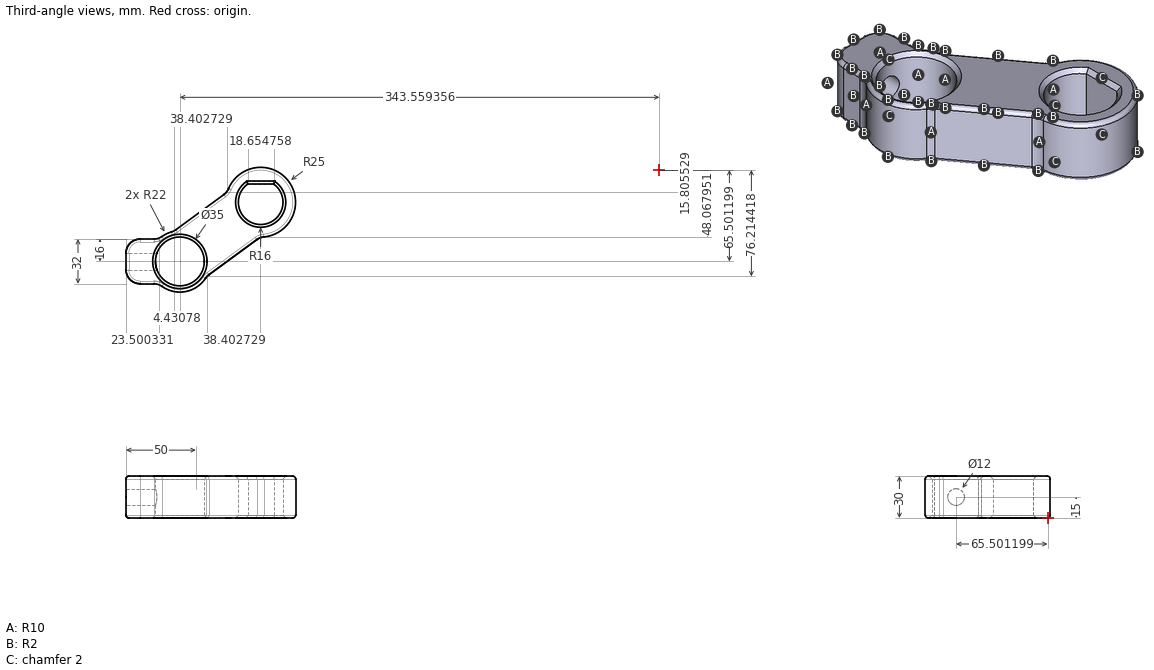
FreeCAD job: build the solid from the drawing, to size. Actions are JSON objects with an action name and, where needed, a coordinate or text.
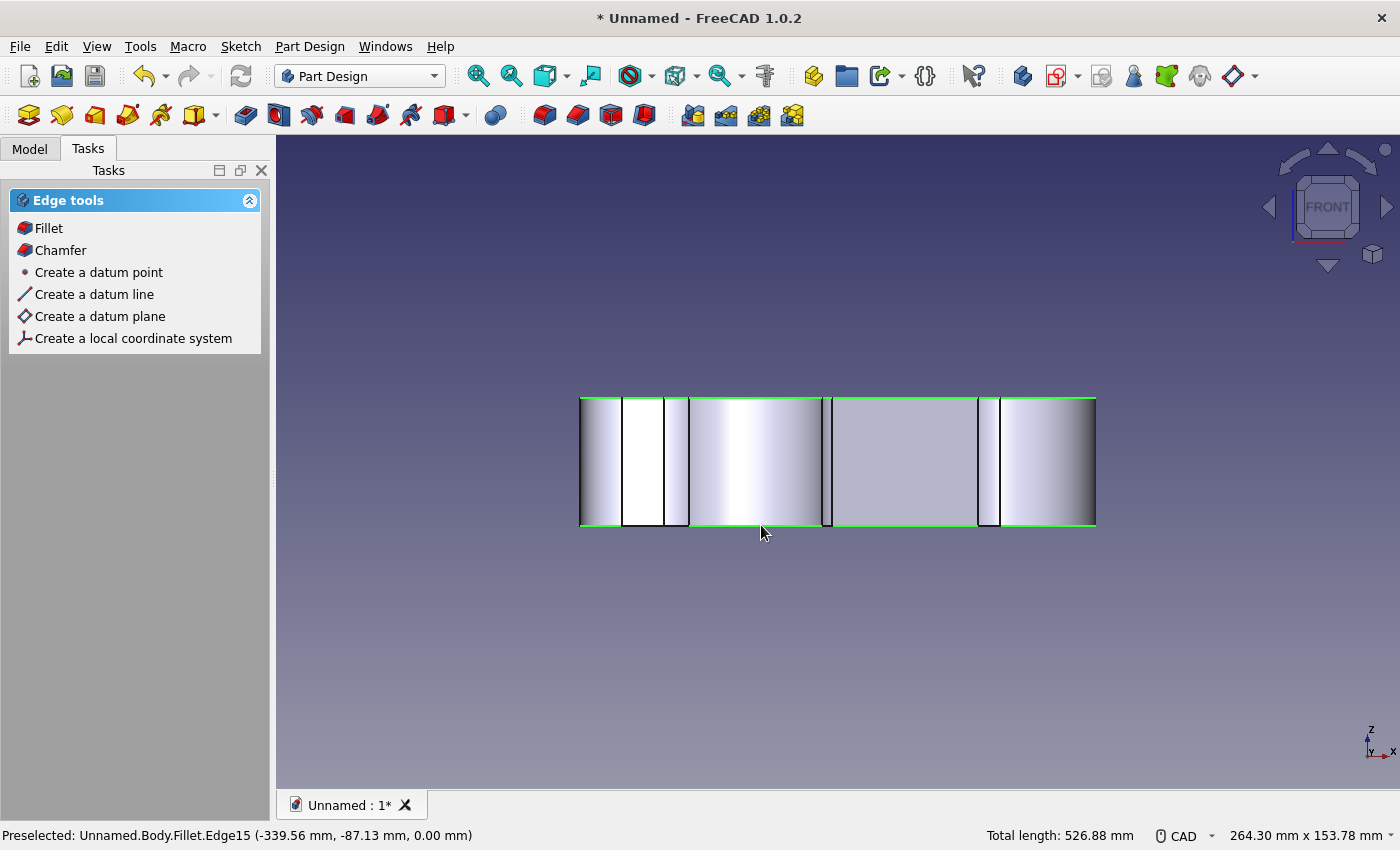
{"action": "left_click", "coordinate": [643, 525], "text": "ctrl"}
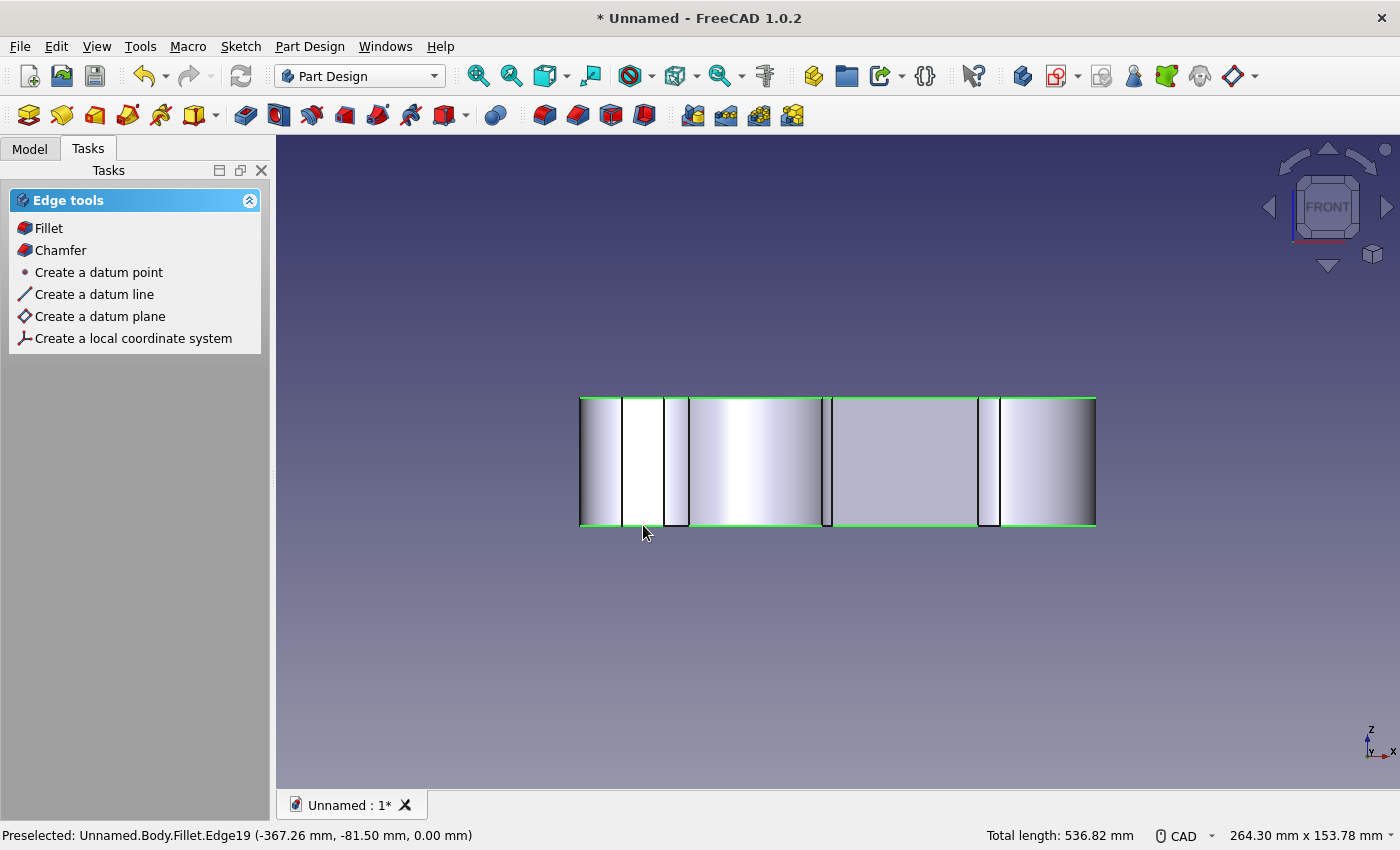
{"action": "left_click", "coordinate": [828, 525], "text": "ctrl"}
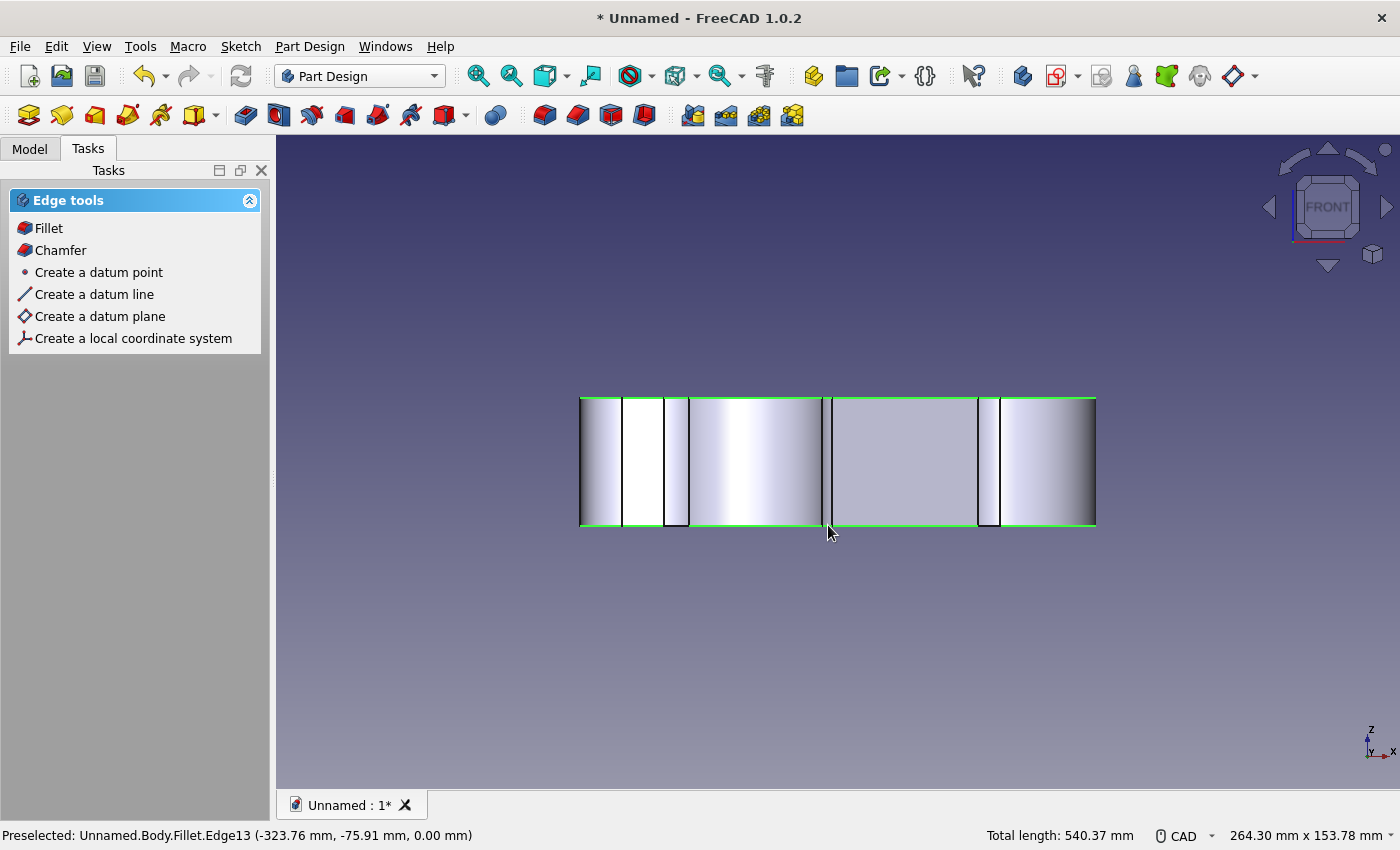
{"action": "left_click", "coordinate": [678, 525], "text": "ctrl"}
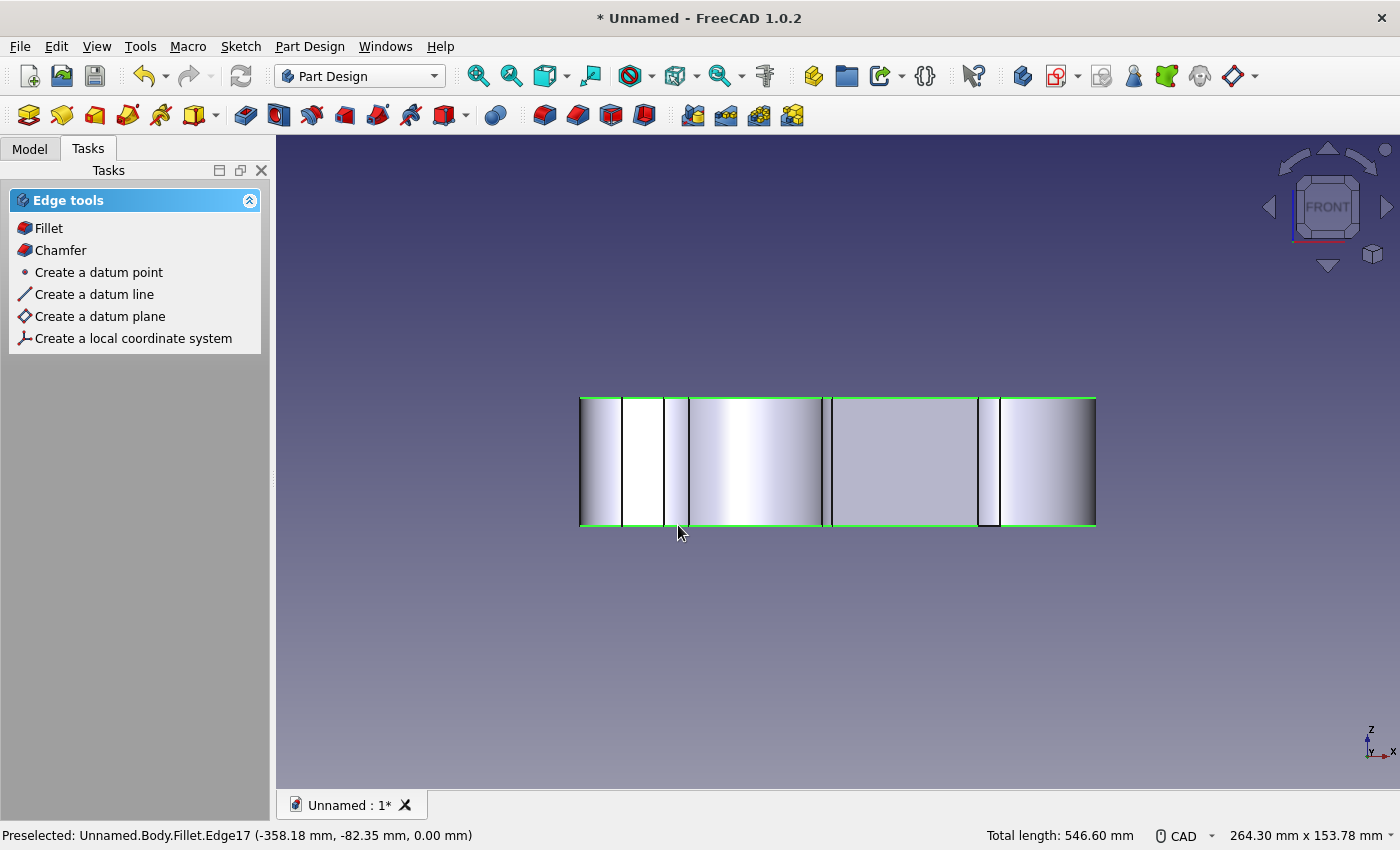
{"action": "left_click", "coordinate": [989, 525], "text": "ctrl"}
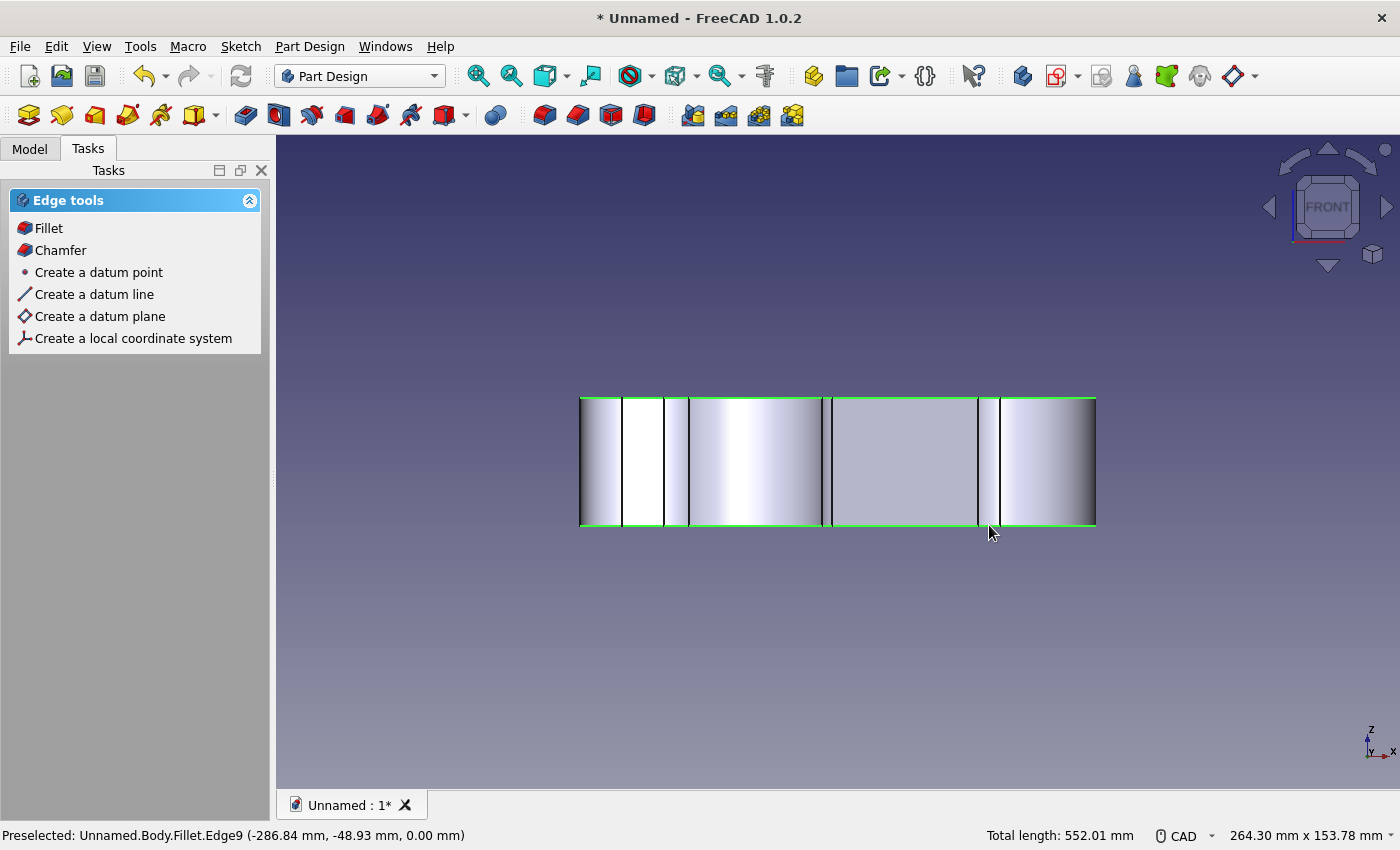
{"action": "key", "text": "3"}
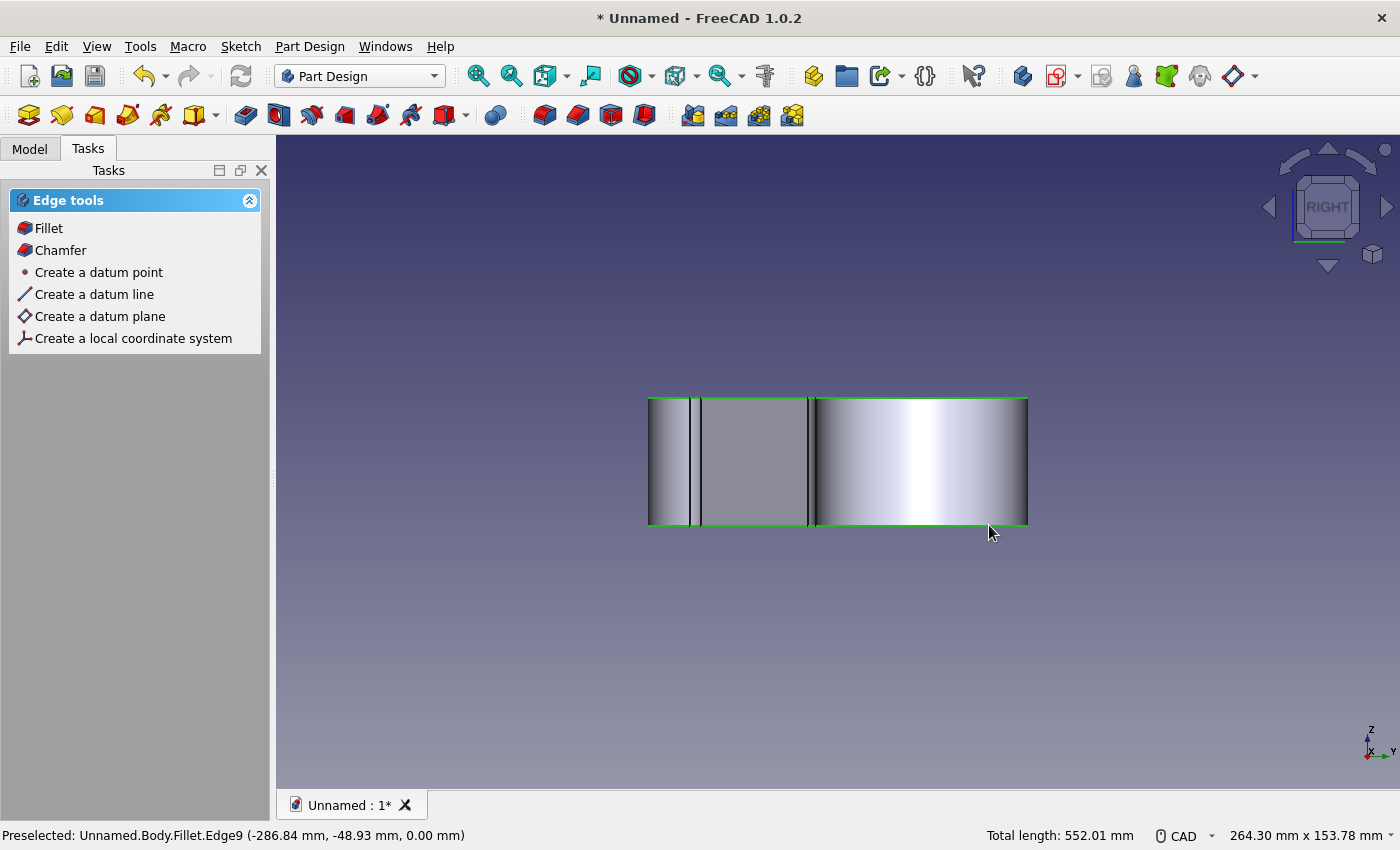
{"action": "left_click", "coordinate": [479, 76]}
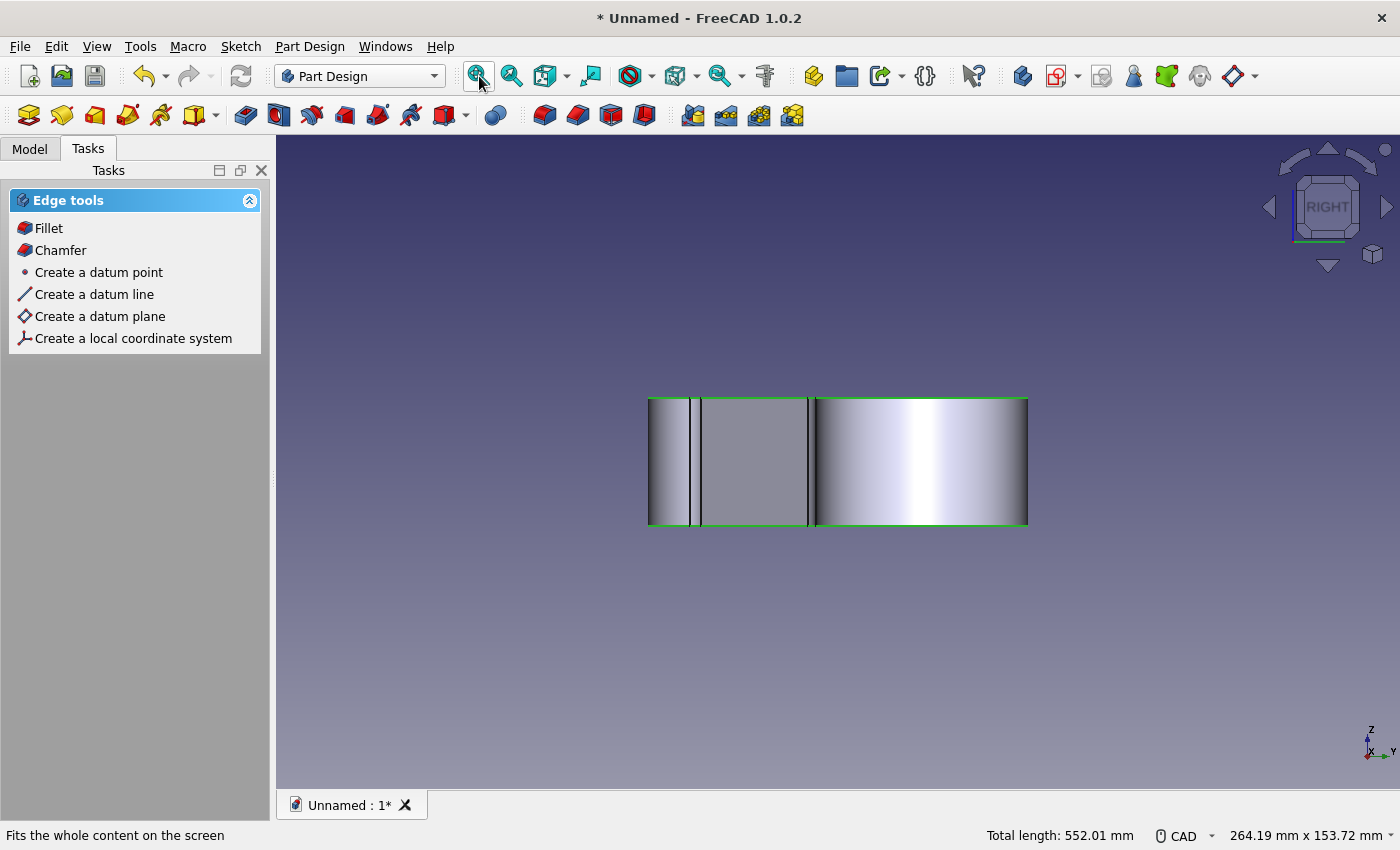
{"action": "key", "text": "5"}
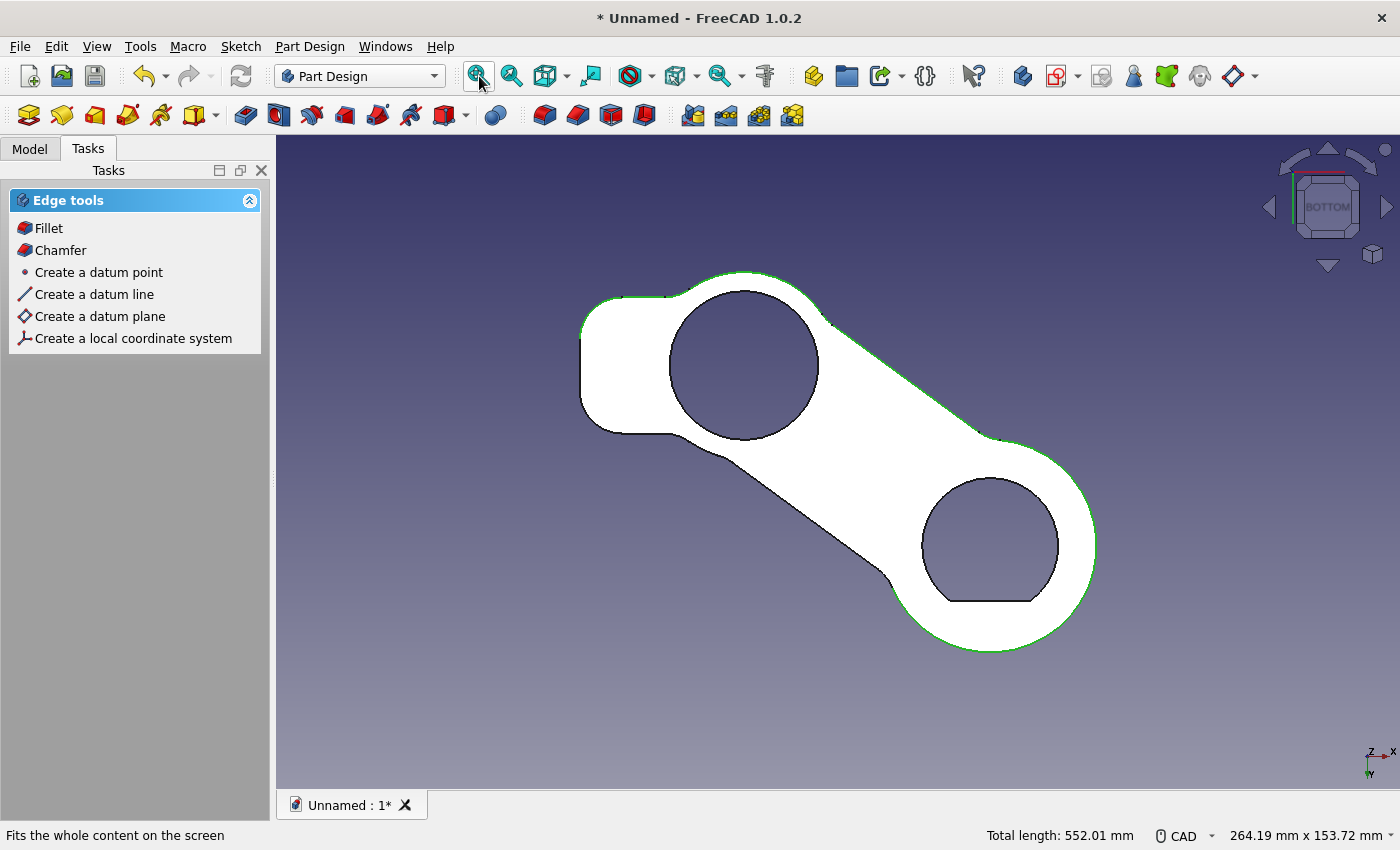
{"action": "left_click", "coordinate": [703, 449], "text": "ctrl"}